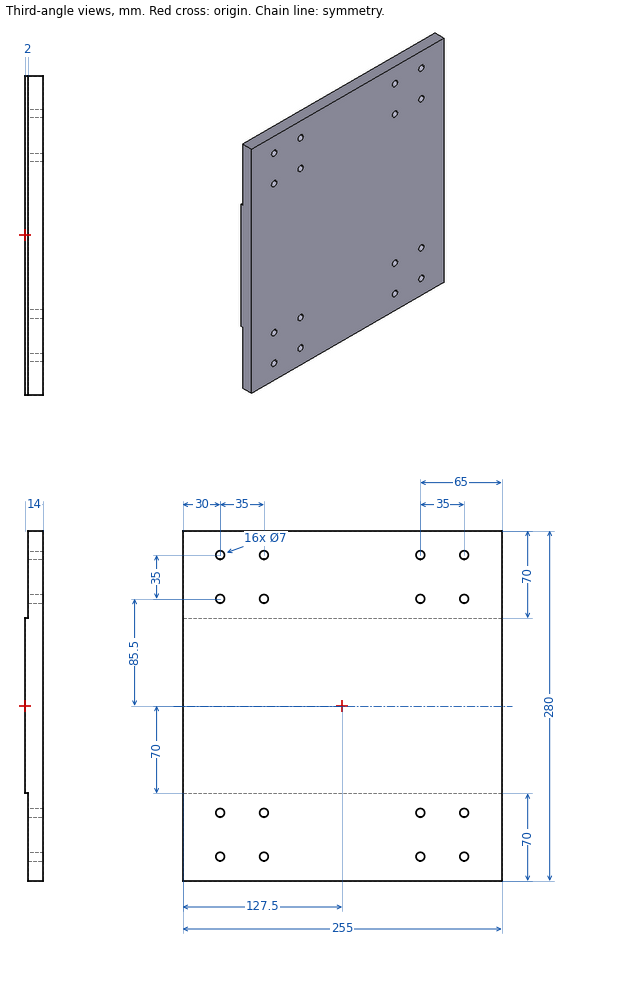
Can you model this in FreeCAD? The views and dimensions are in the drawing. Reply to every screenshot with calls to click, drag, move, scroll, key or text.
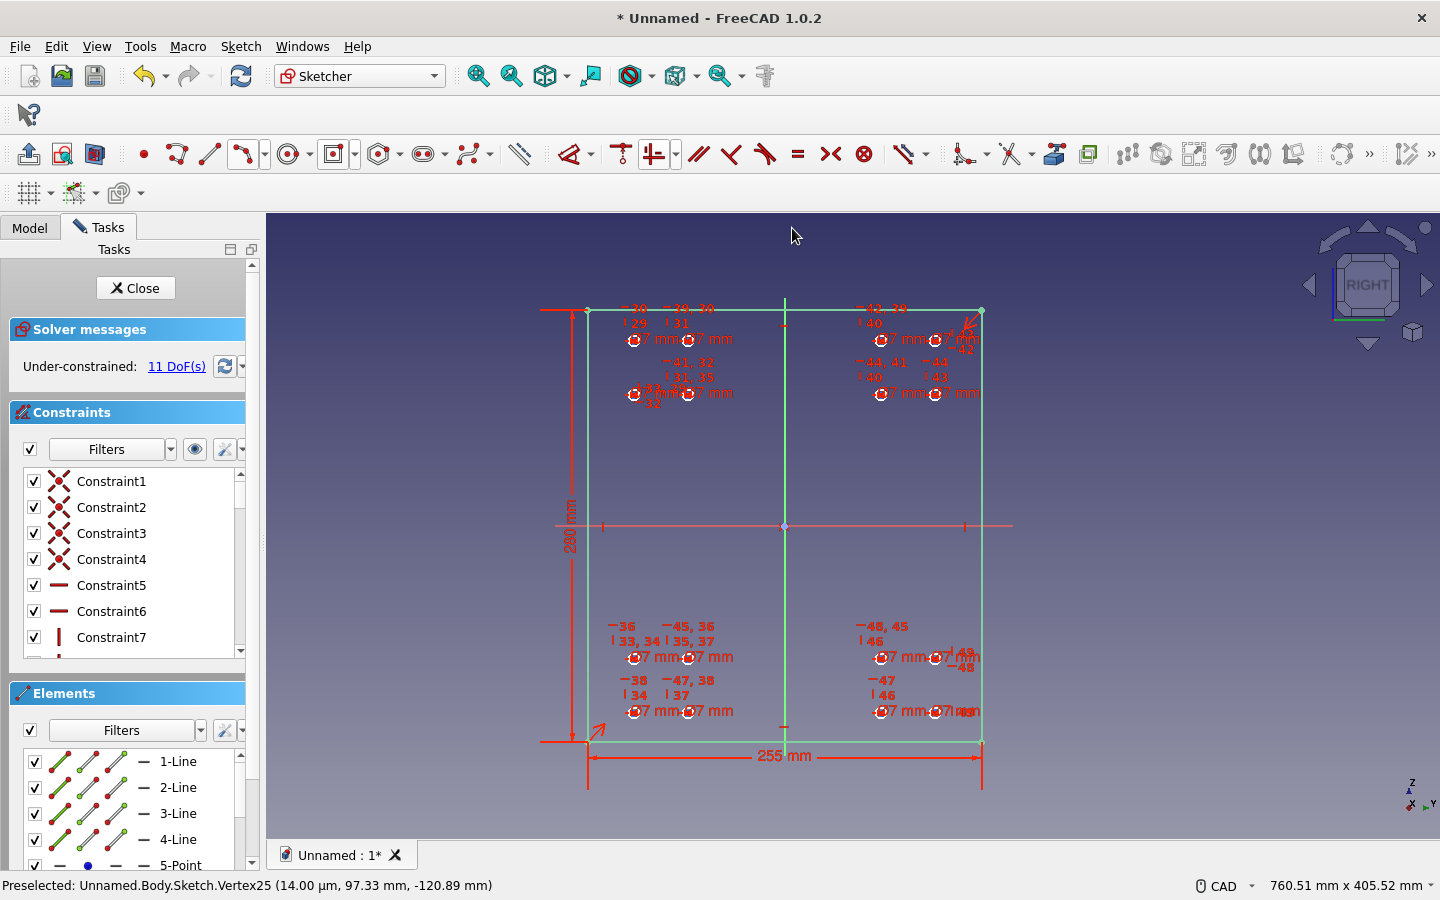
click(881, 713)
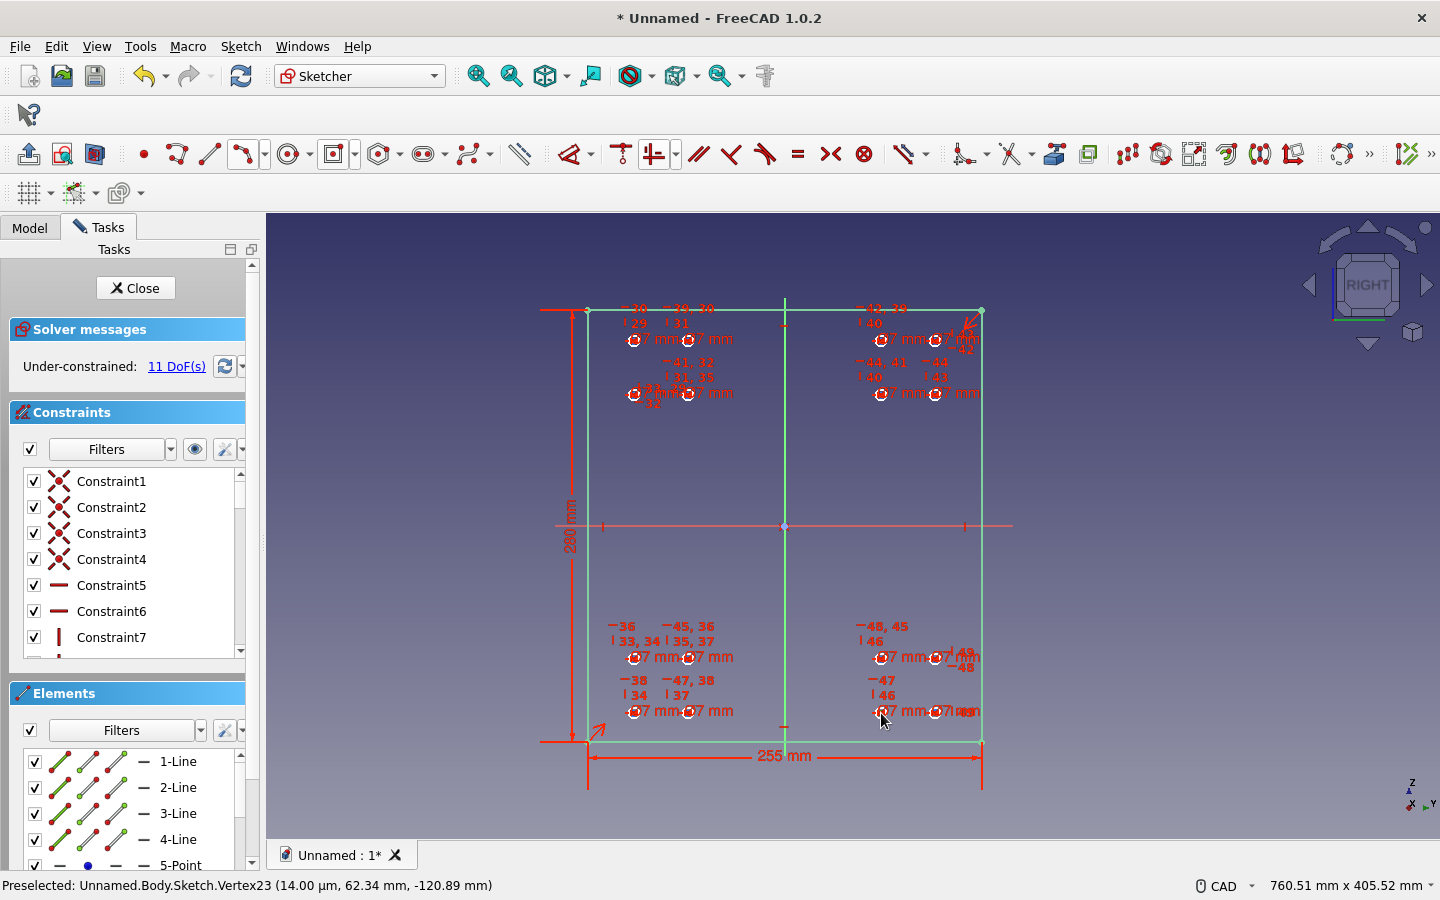
click(935, 713)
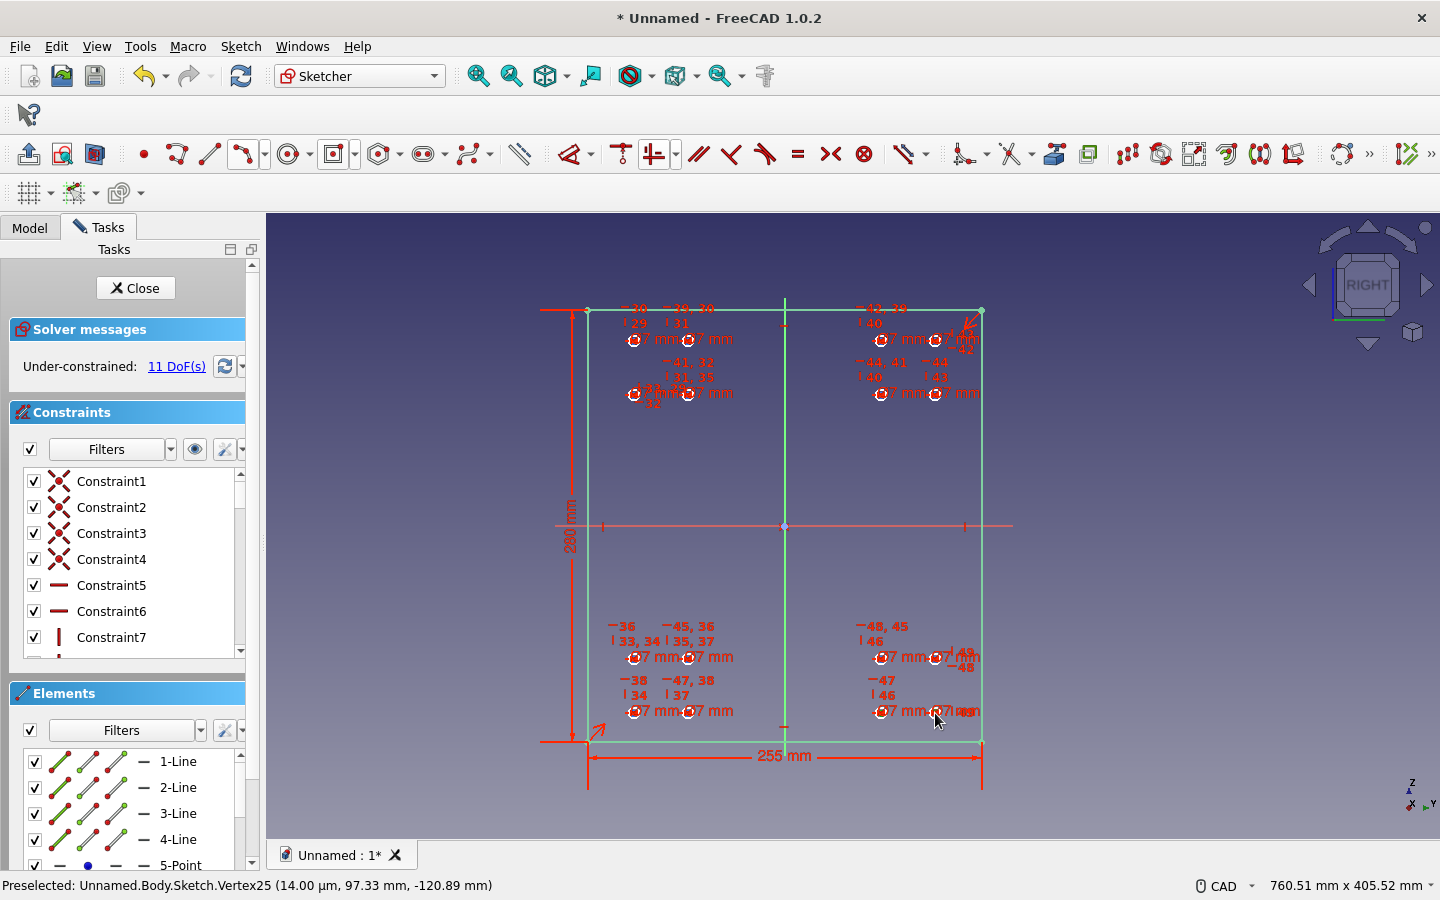
key(h)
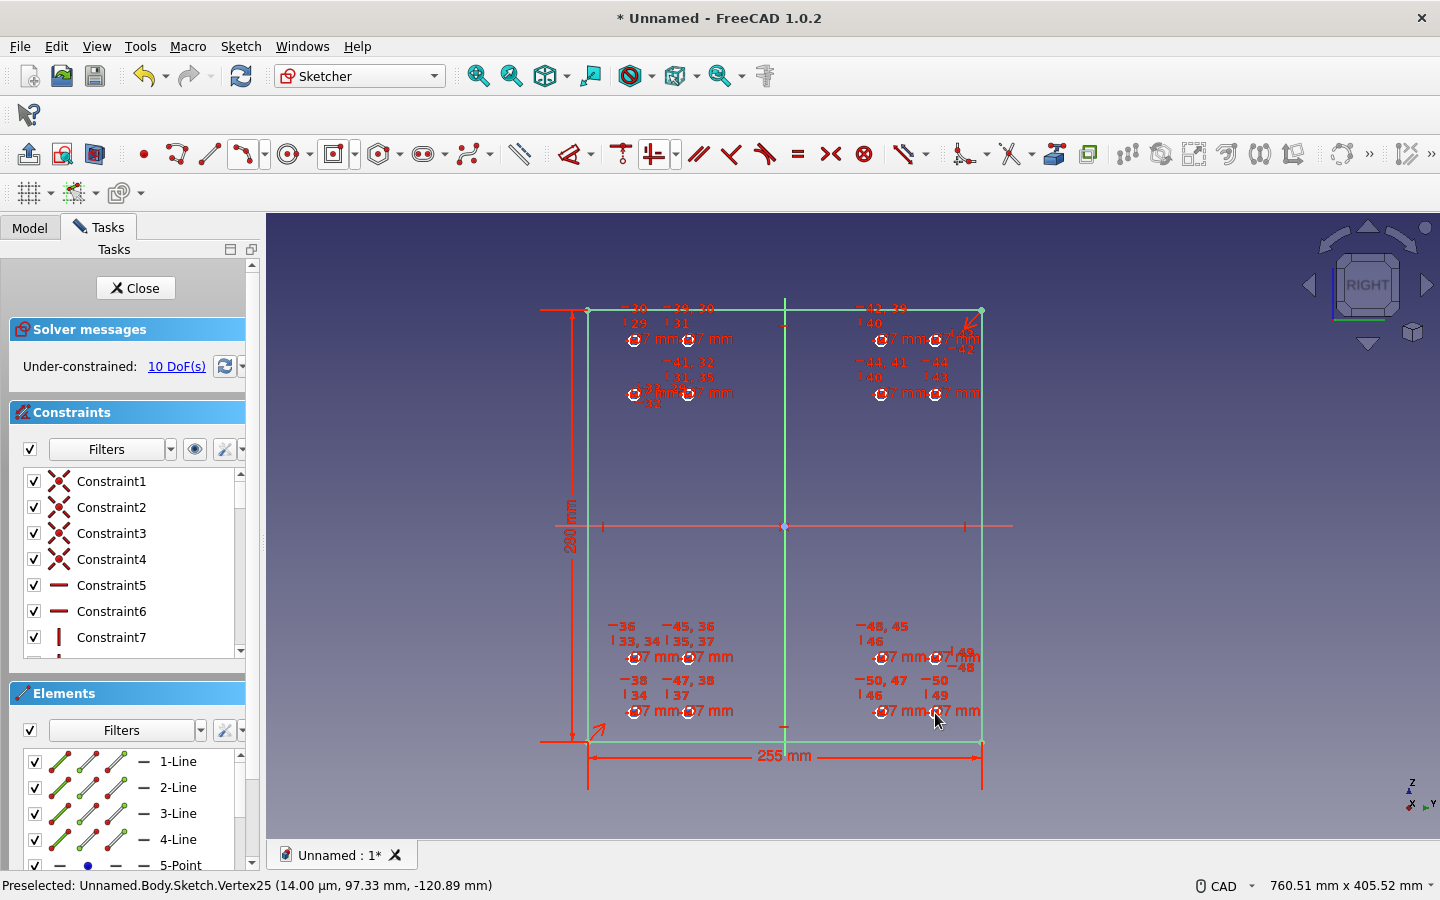
click(881, 395)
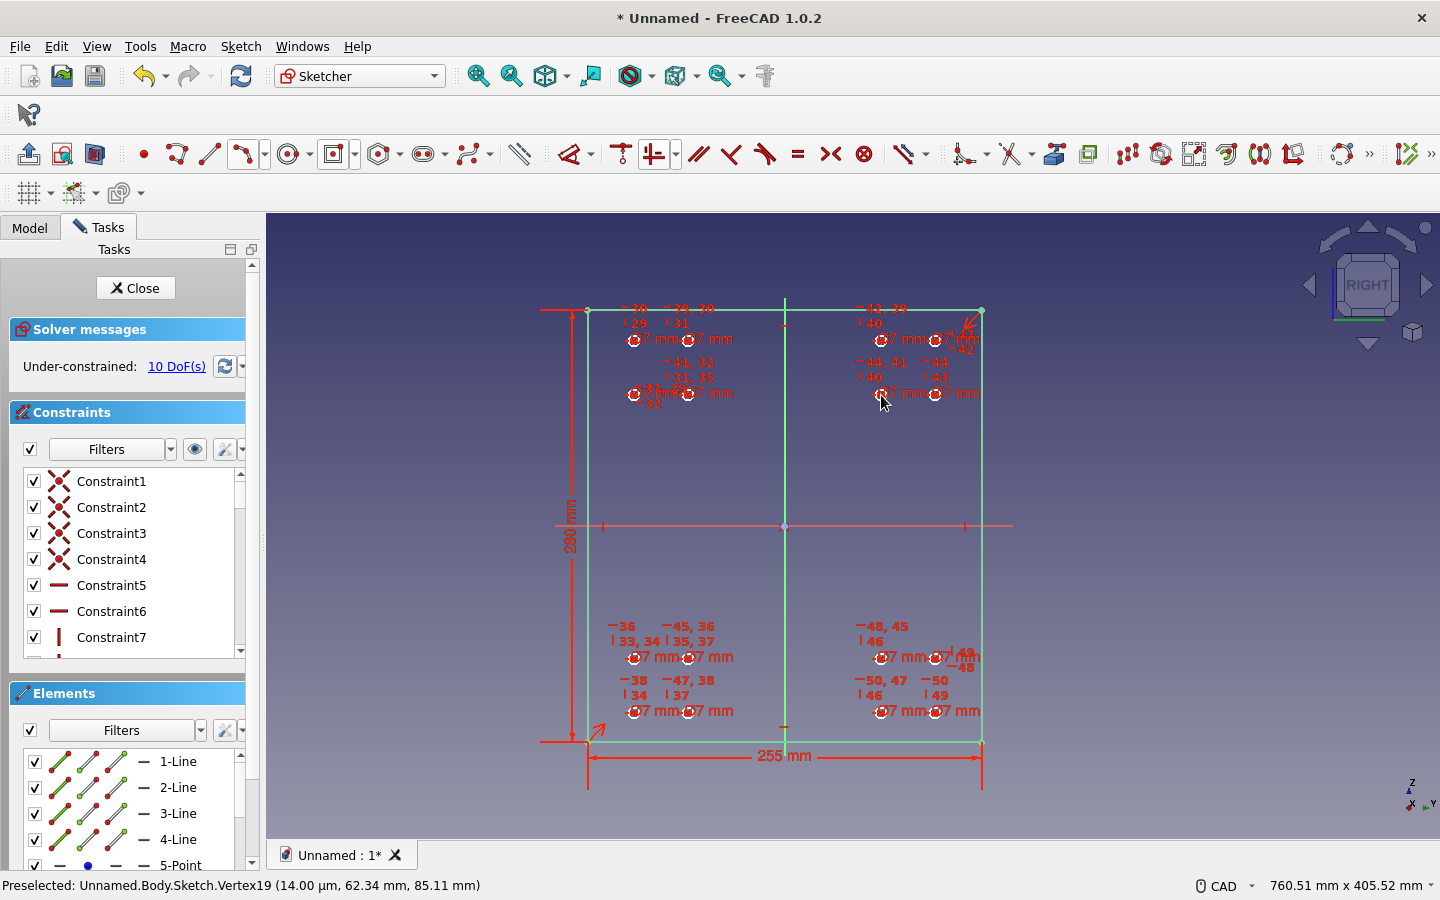
click(881, 659)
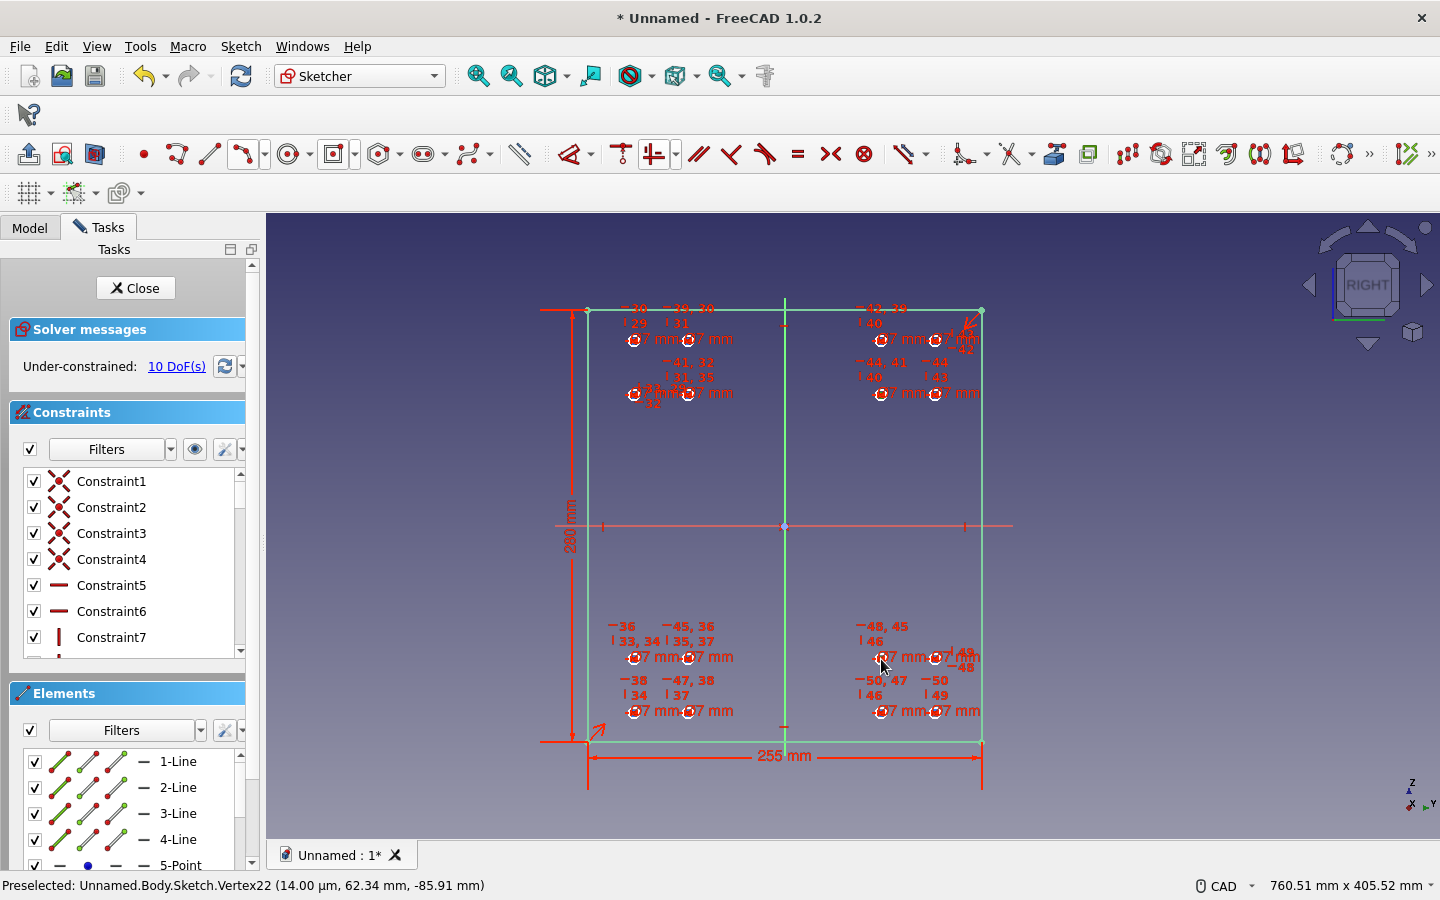
click(644, 526)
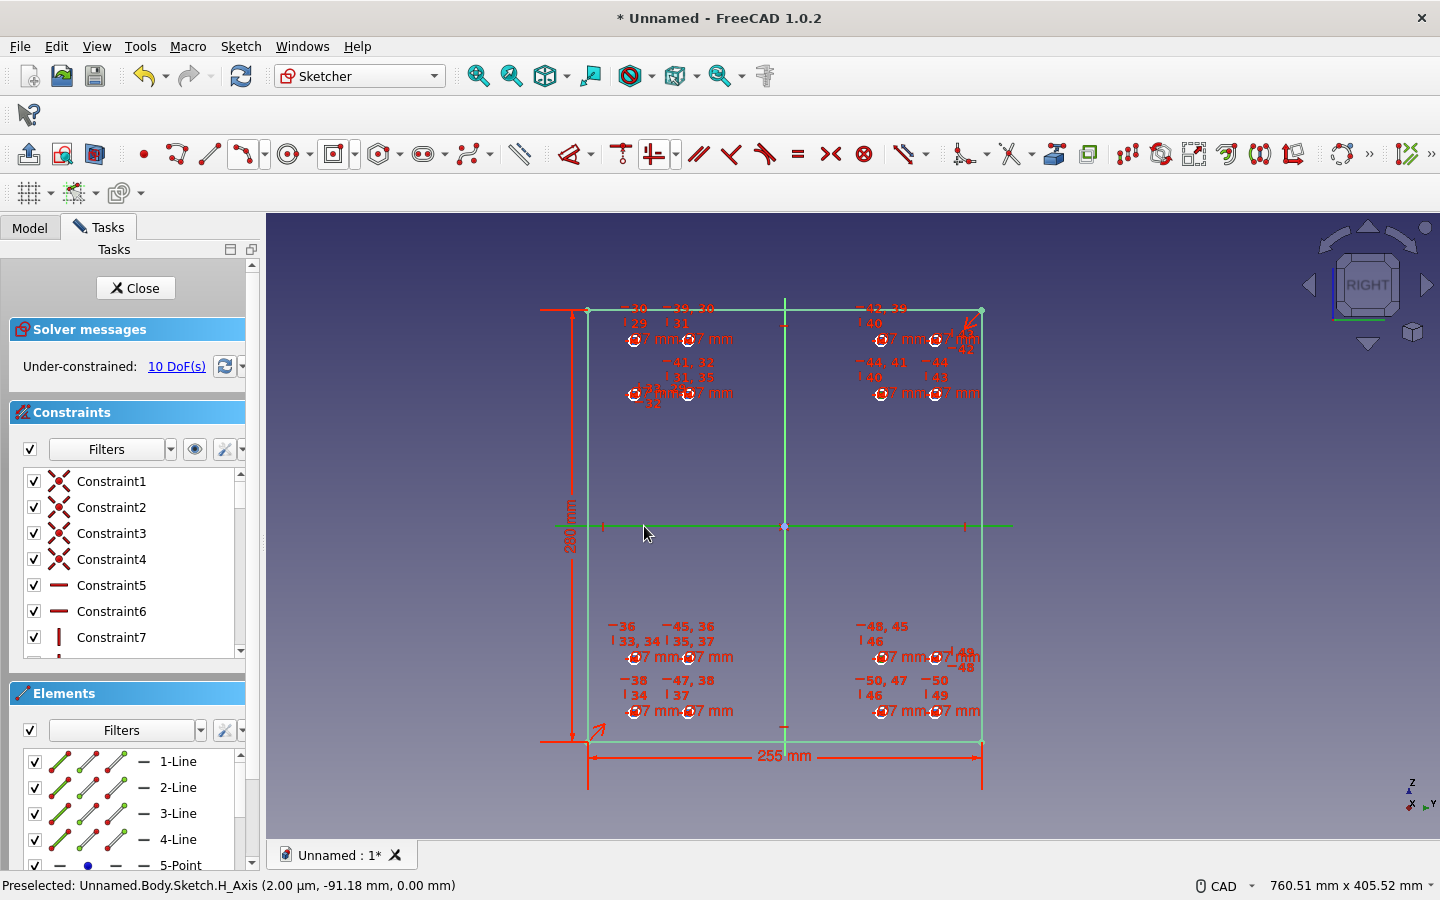
click(831, 154)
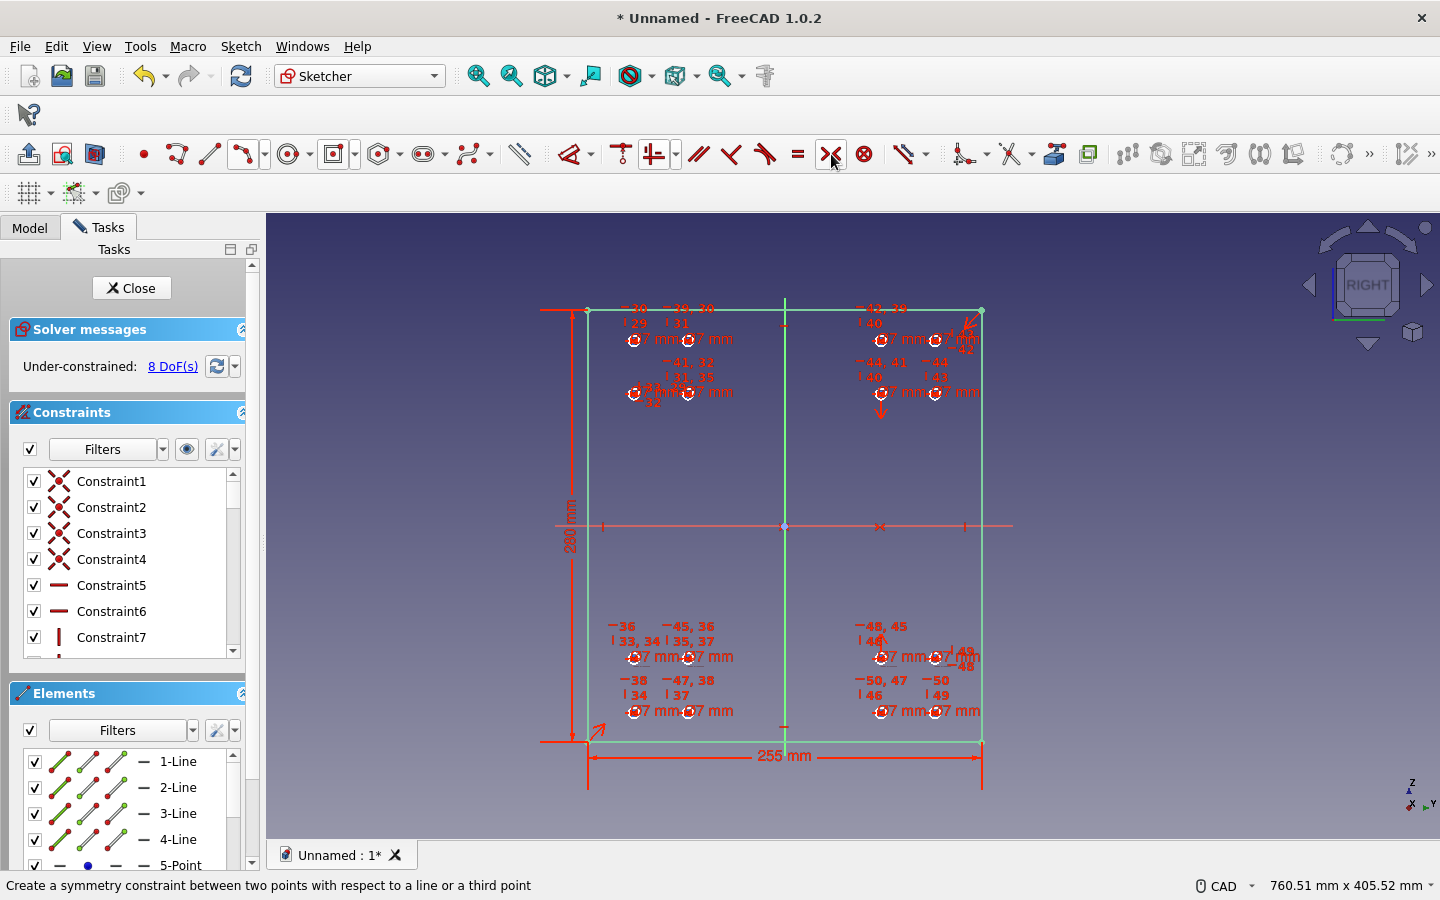
click(935, 341)